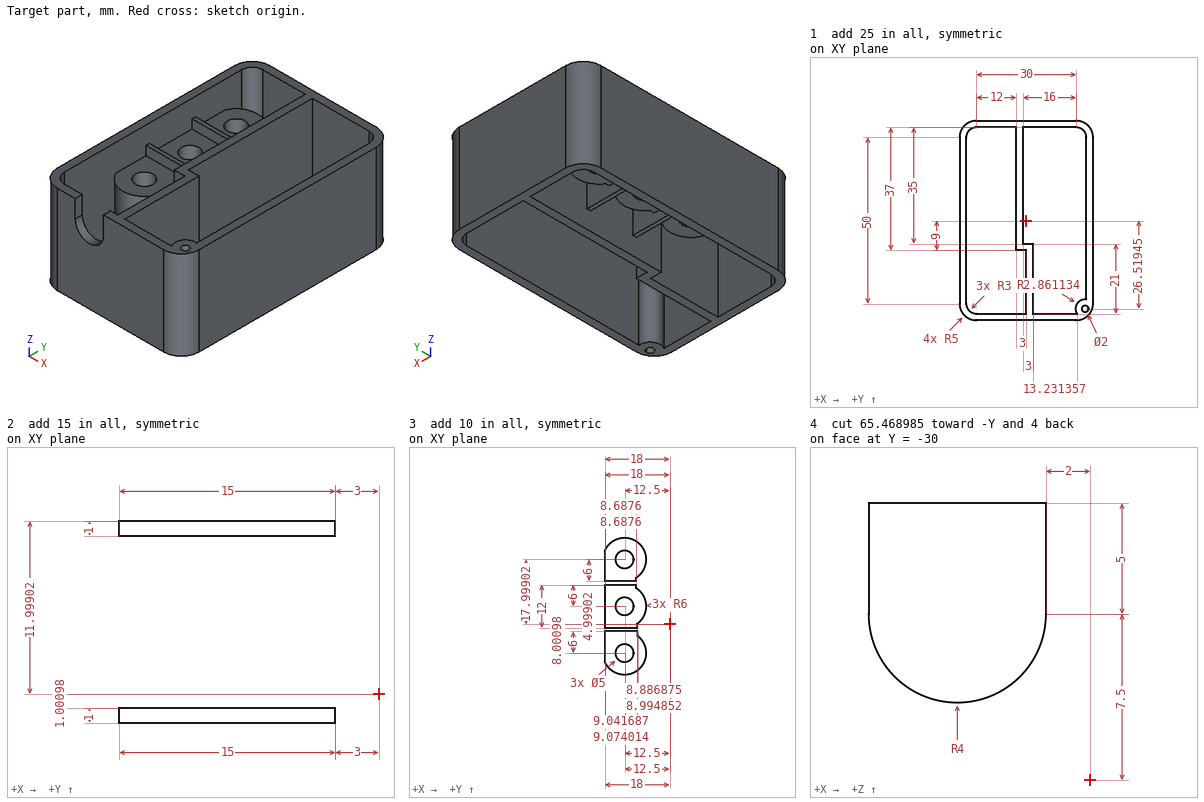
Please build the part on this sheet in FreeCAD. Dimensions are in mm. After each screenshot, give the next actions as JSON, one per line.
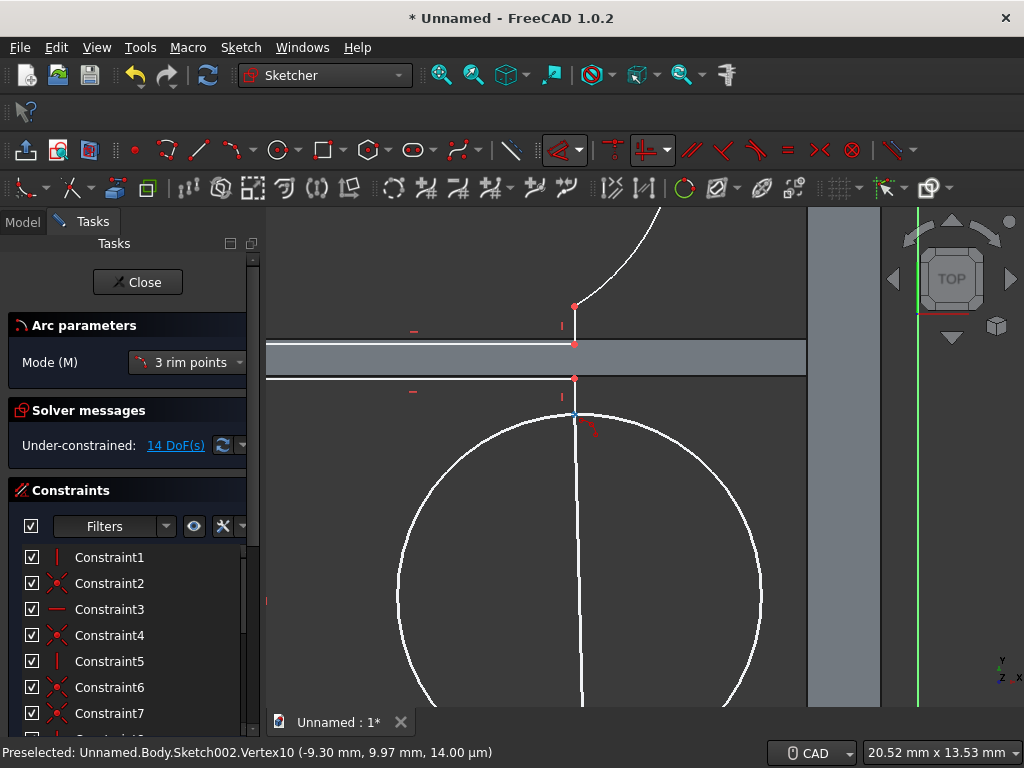
{"action": "scroll", "coordinate": [573, 410], "scroll_direction": "down", "scroll_amount": 7}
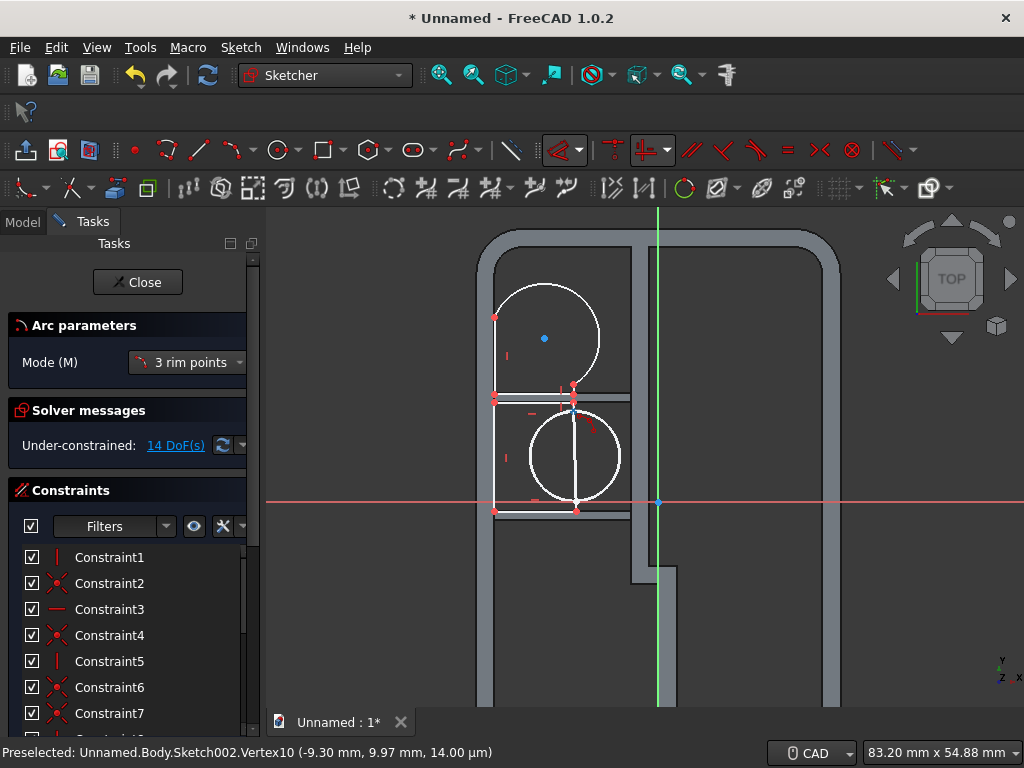
{"action": "left_click", "coordinate": [599, 455]}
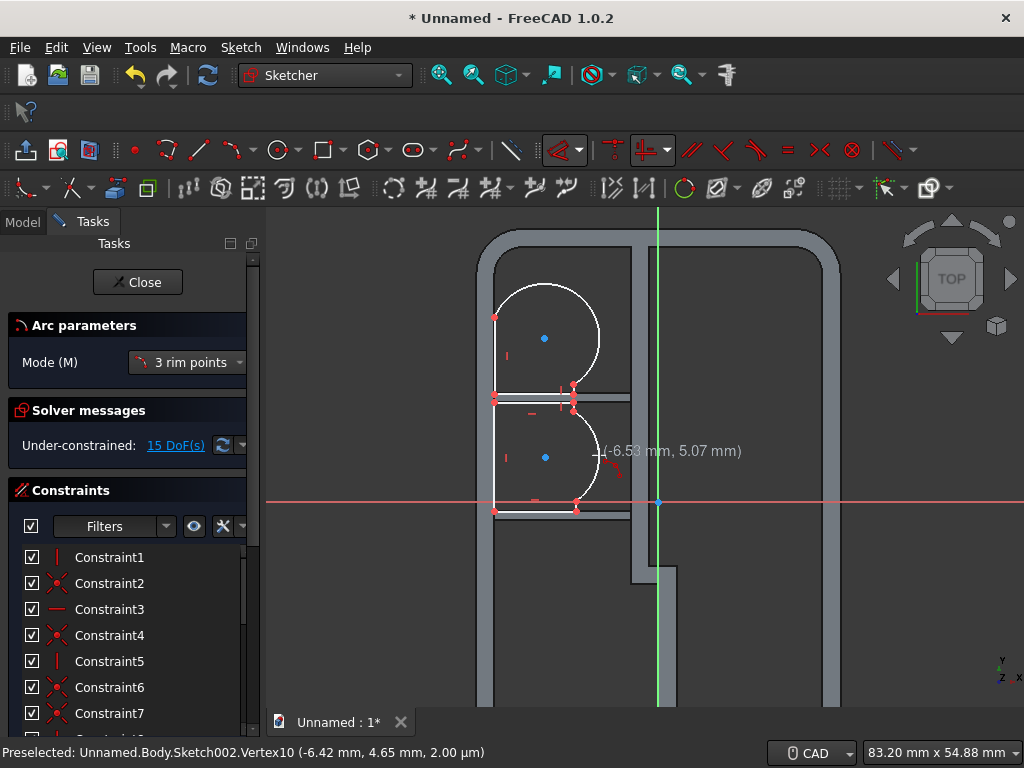
{"action": "left_click", "coordinate": [168, 150]}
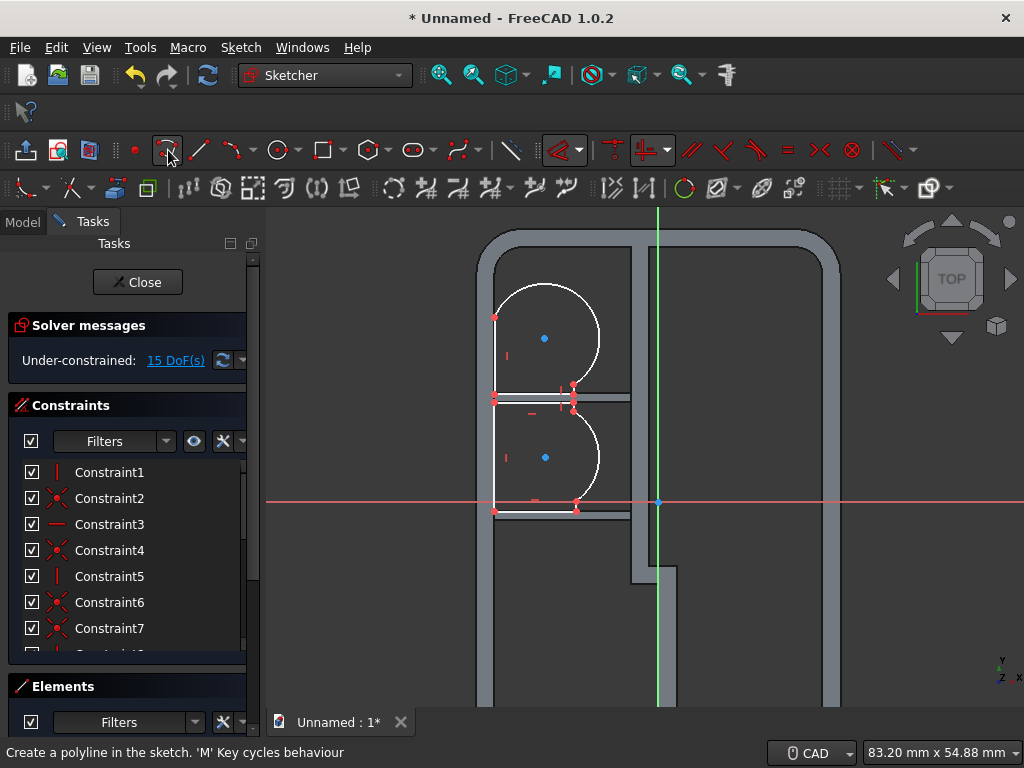
{"action": "left_click", "coordinate": [577, 531]}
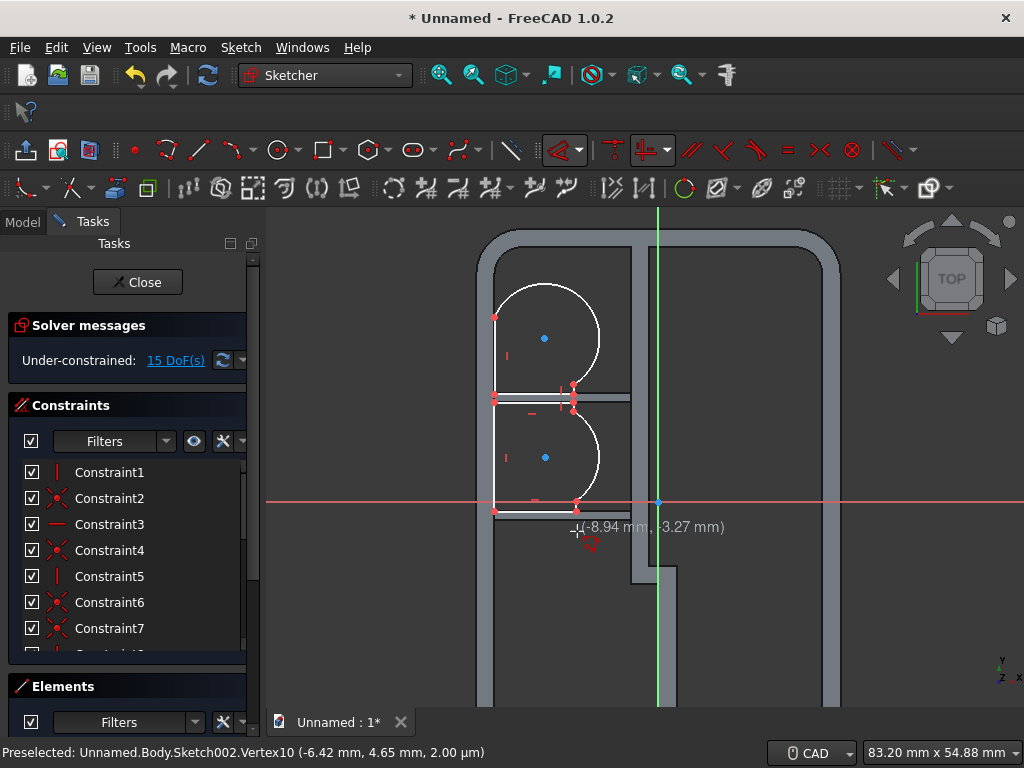
{"action": "scroll", "coordinate": [577, 520], "scroll_direction": "up", "scroll_amount": 3}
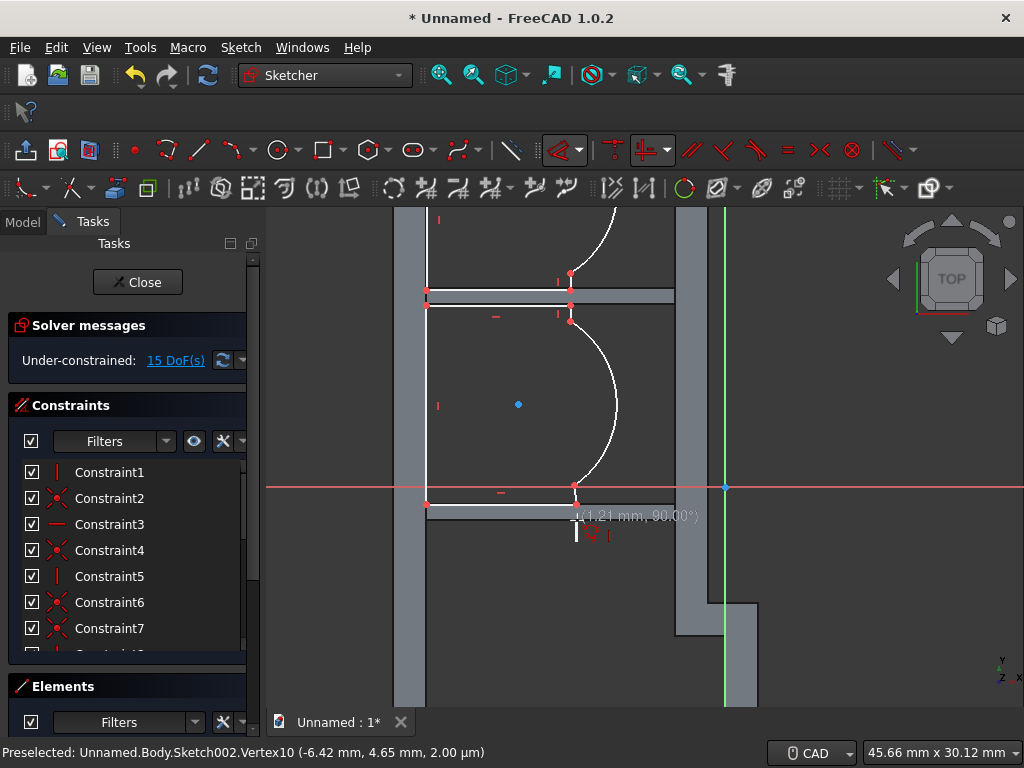
{"action": "left_click", "coordinate": [574, 520]}
{"action": "left_click", "coordinate": [426, 520]}
{"action": "left_click", "coordinate": [426, 660]}
{"action": "right_click", "coordinate": [426, 660]}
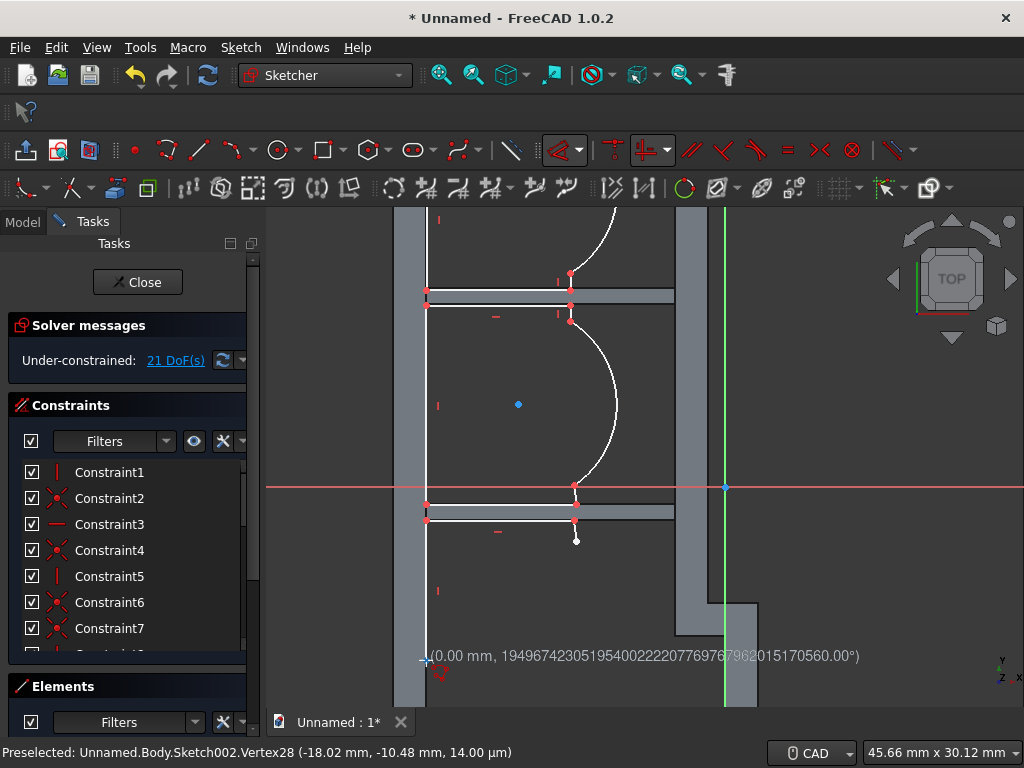
{"action": "left_click", "coordinate": [232, 150]}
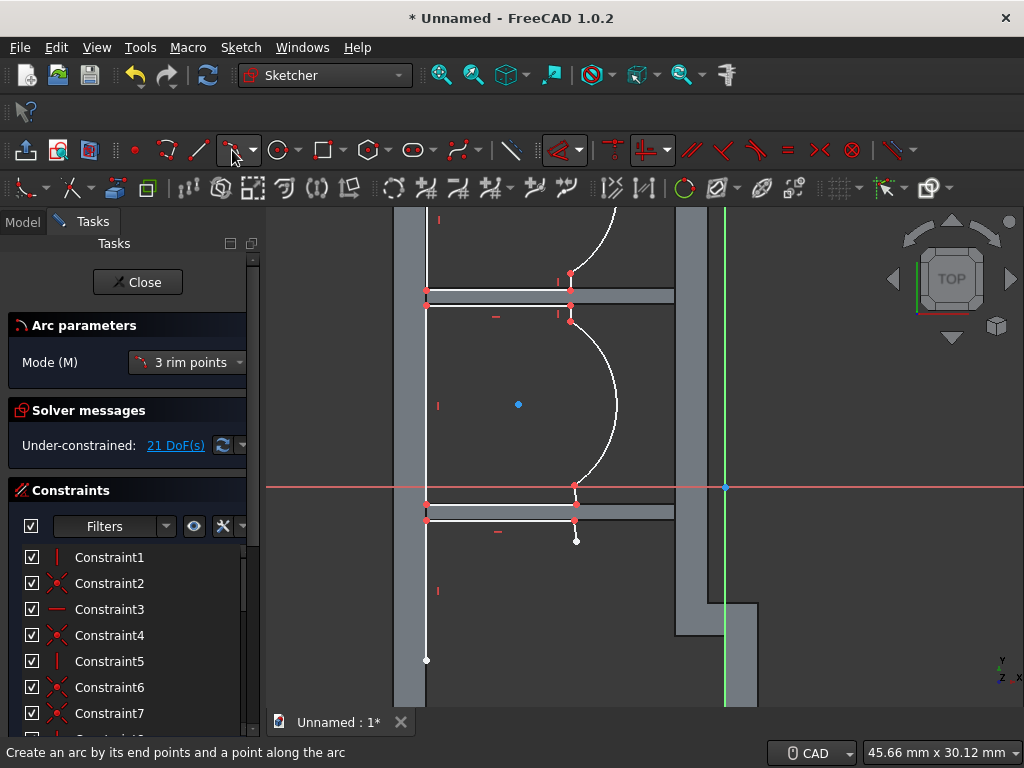
{"action": "left_click", "coordinate": [426, 661]}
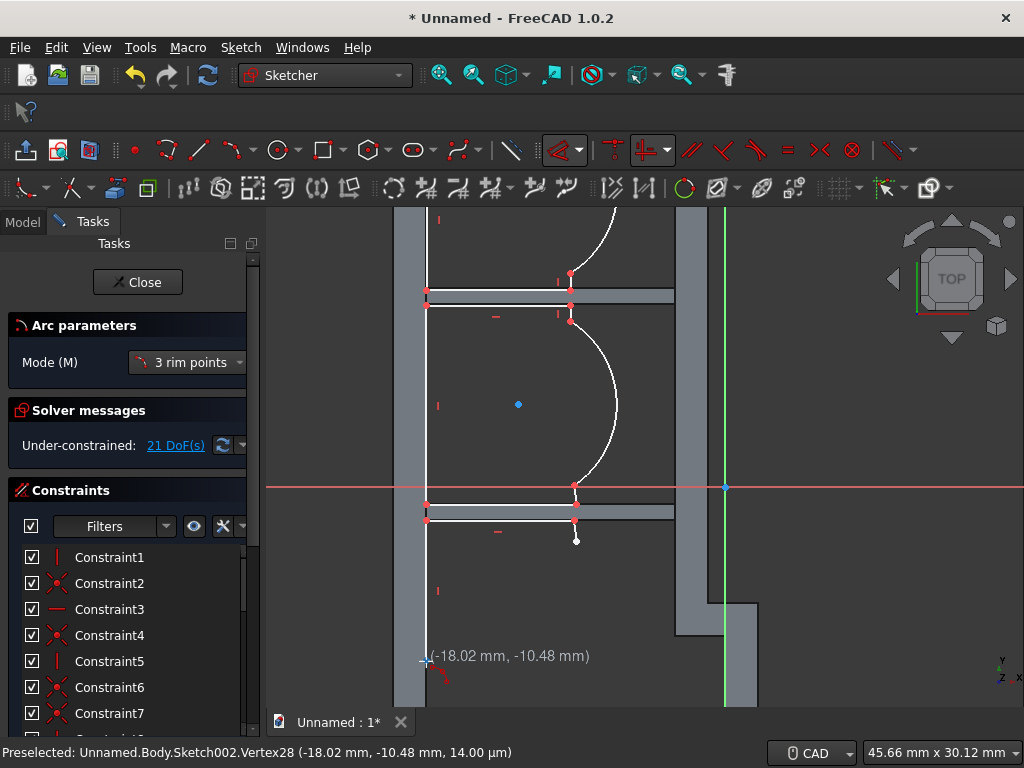
{"action": "scroll", "coordinate": [578, 540], "scroll_direction": "up", "scroll_amount": 3}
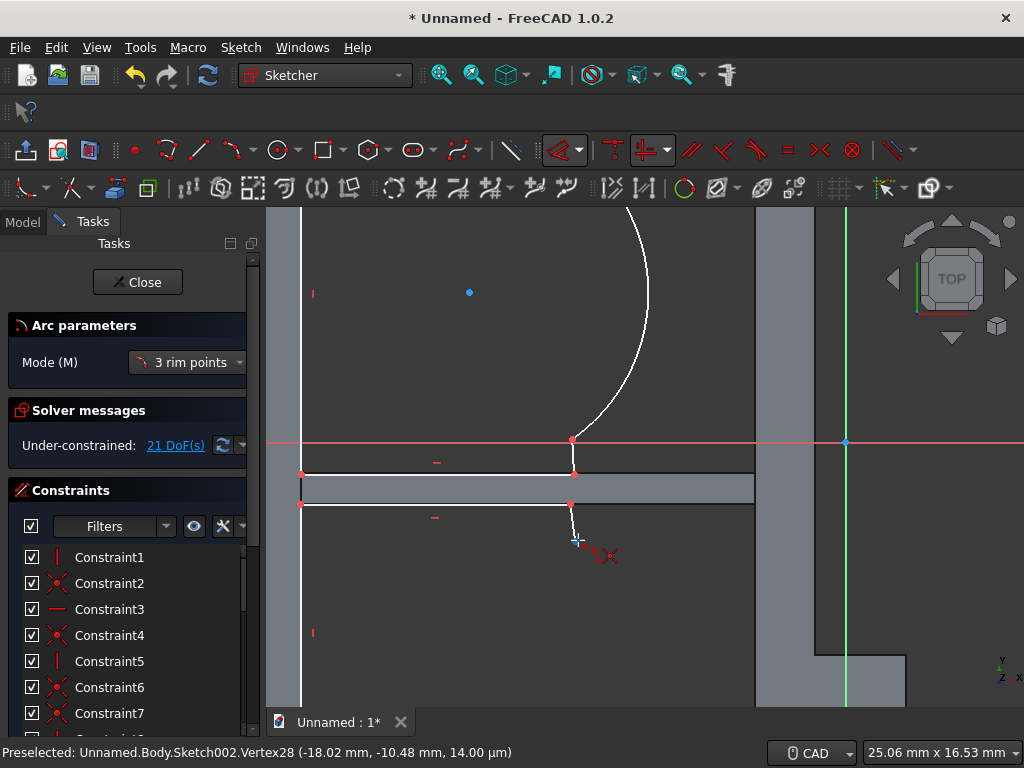
{"action": "left_click", "coordinate": [575, 542]}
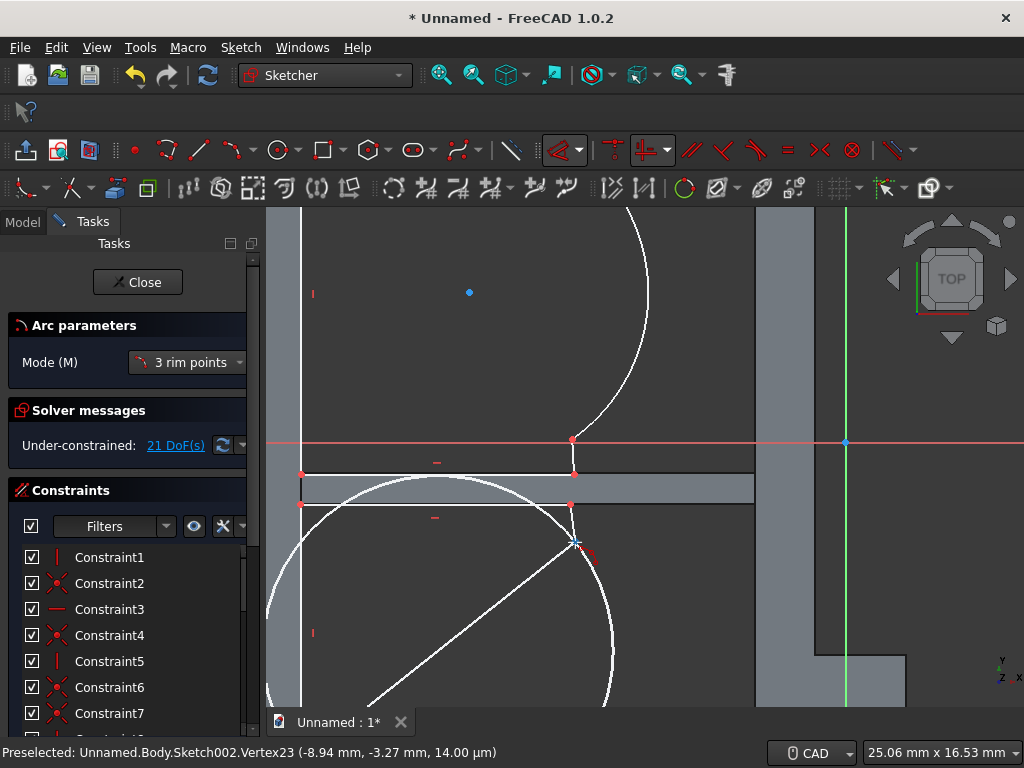
{"action": "scroll", "coordinate": [578, 527], "scroll_direction": "down", "scroll_amount": 6}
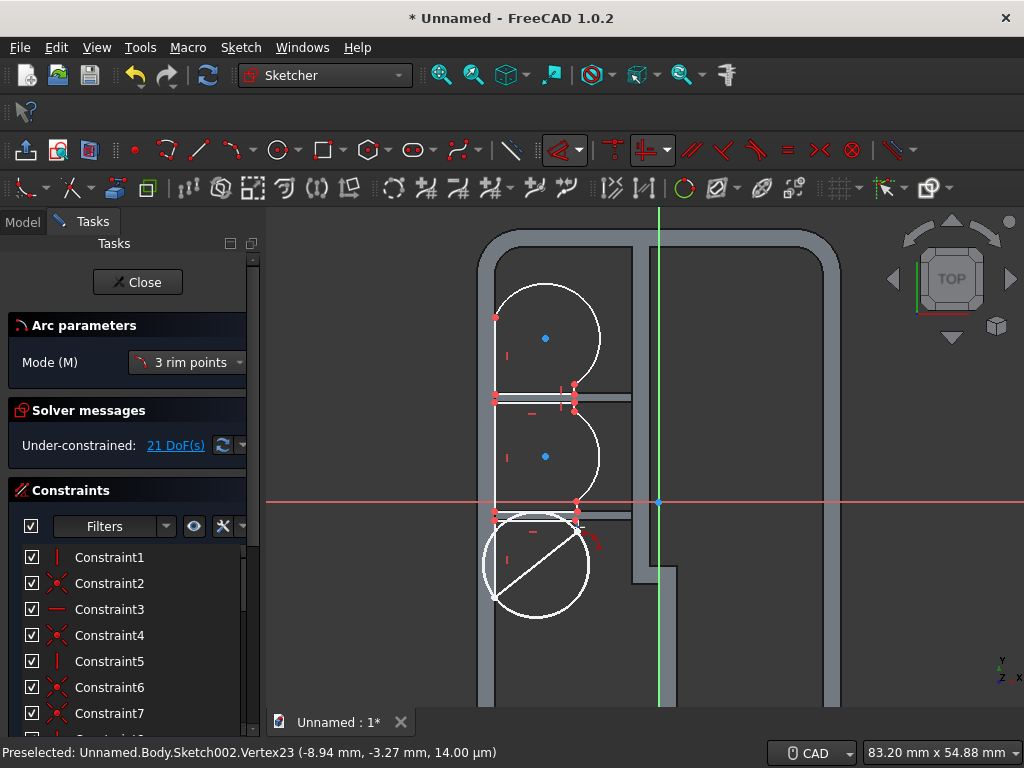
{"action": "left_click", "coordinate": [579, 618]}